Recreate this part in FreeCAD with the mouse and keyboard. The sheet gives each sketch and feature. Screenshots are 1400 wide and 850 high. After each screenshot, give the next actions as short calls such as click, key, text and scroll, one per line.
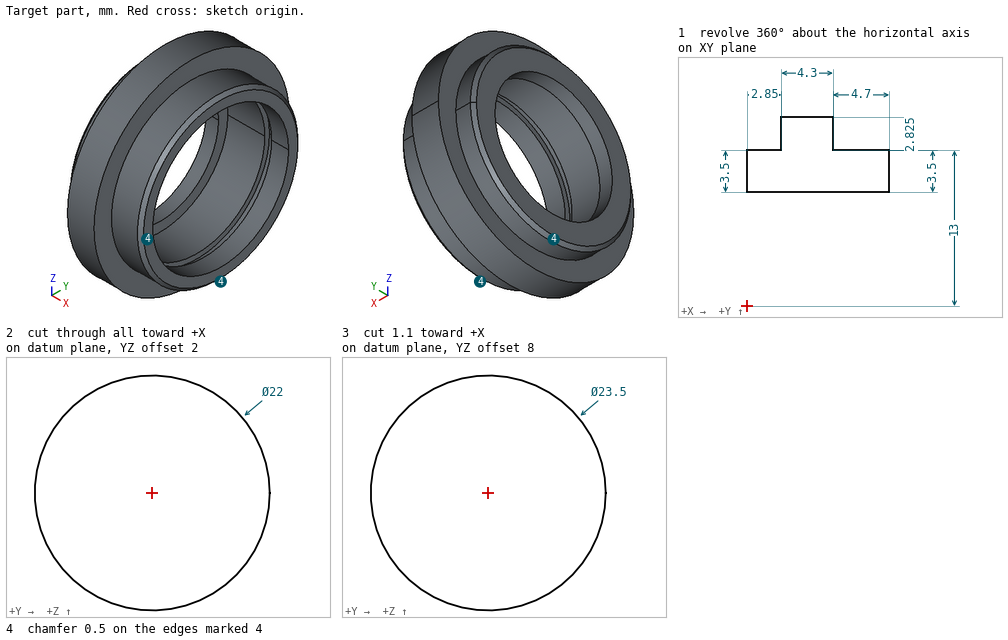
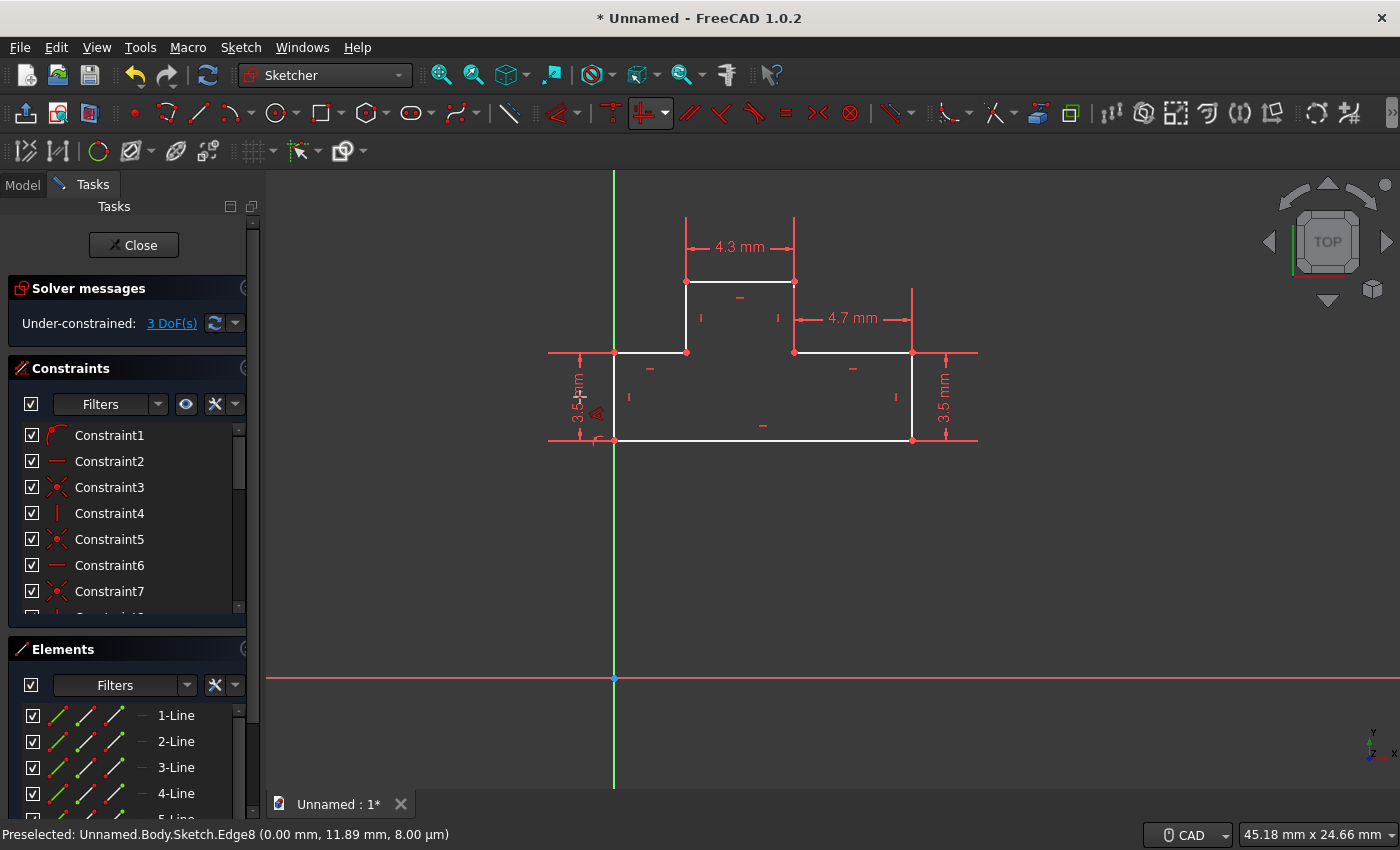
click(912, 353)
click(946, 516)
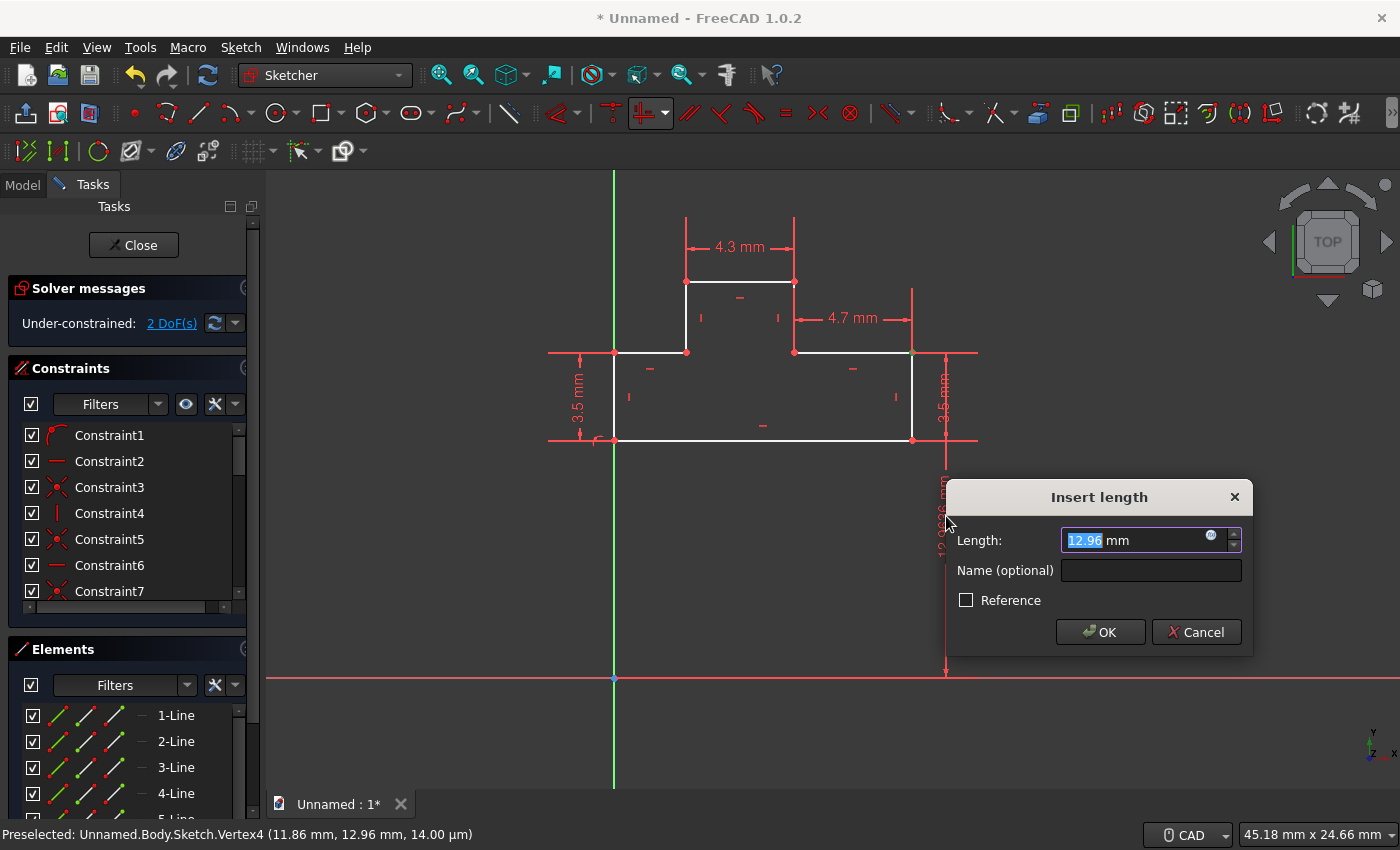
text(13)
key(Return)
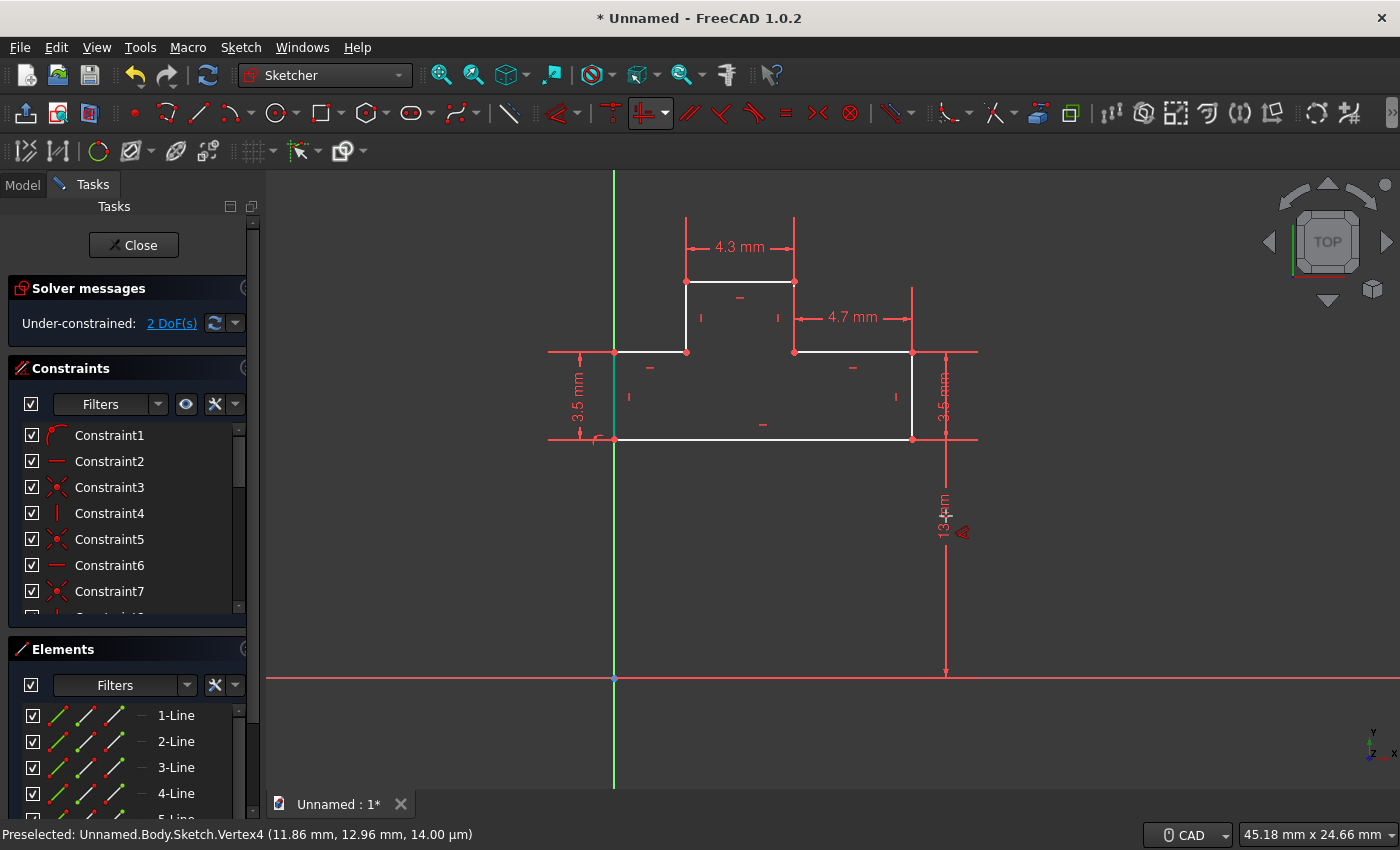
click(665, 352)
click(650, 318)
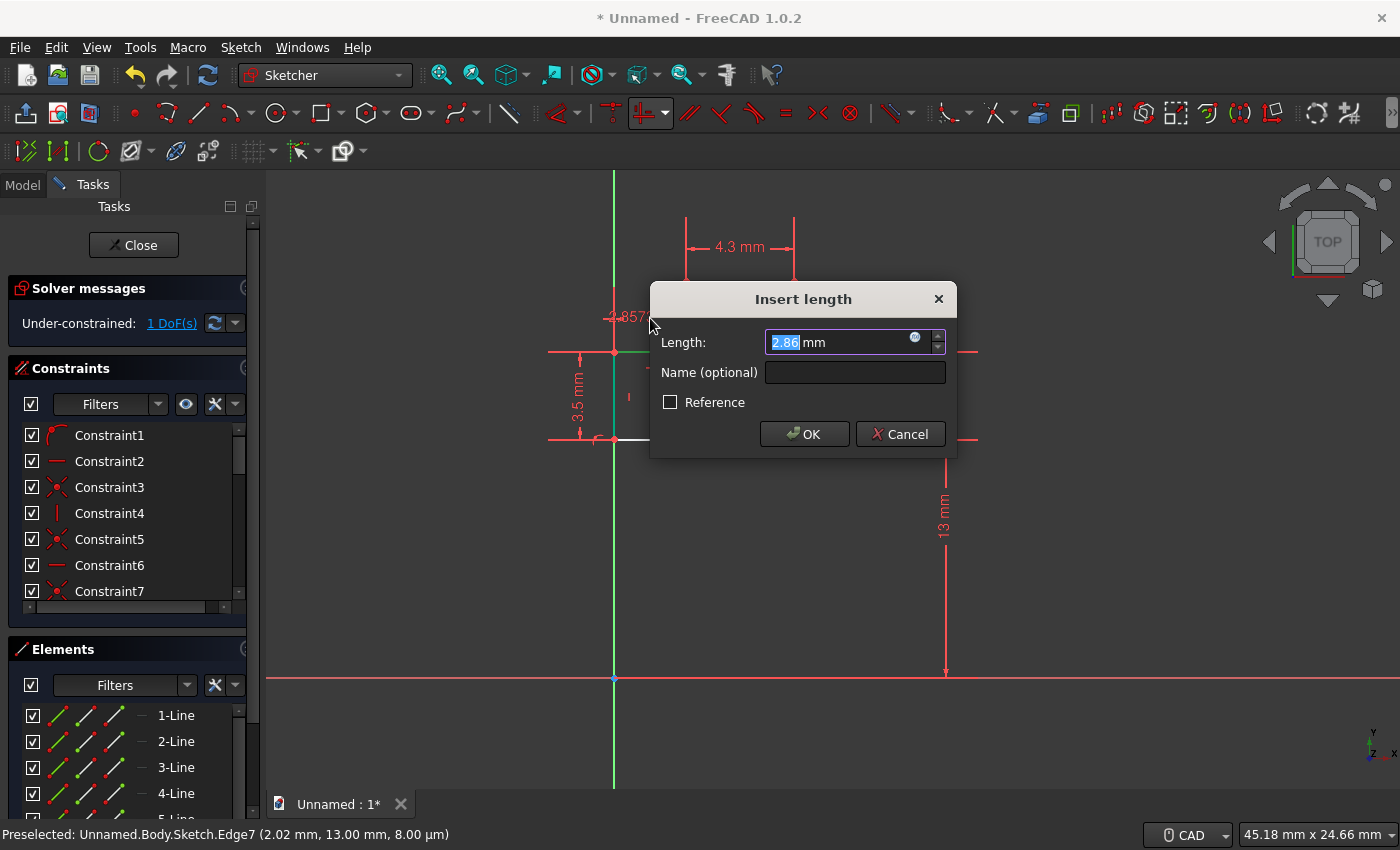
text(2.85)
key(Return)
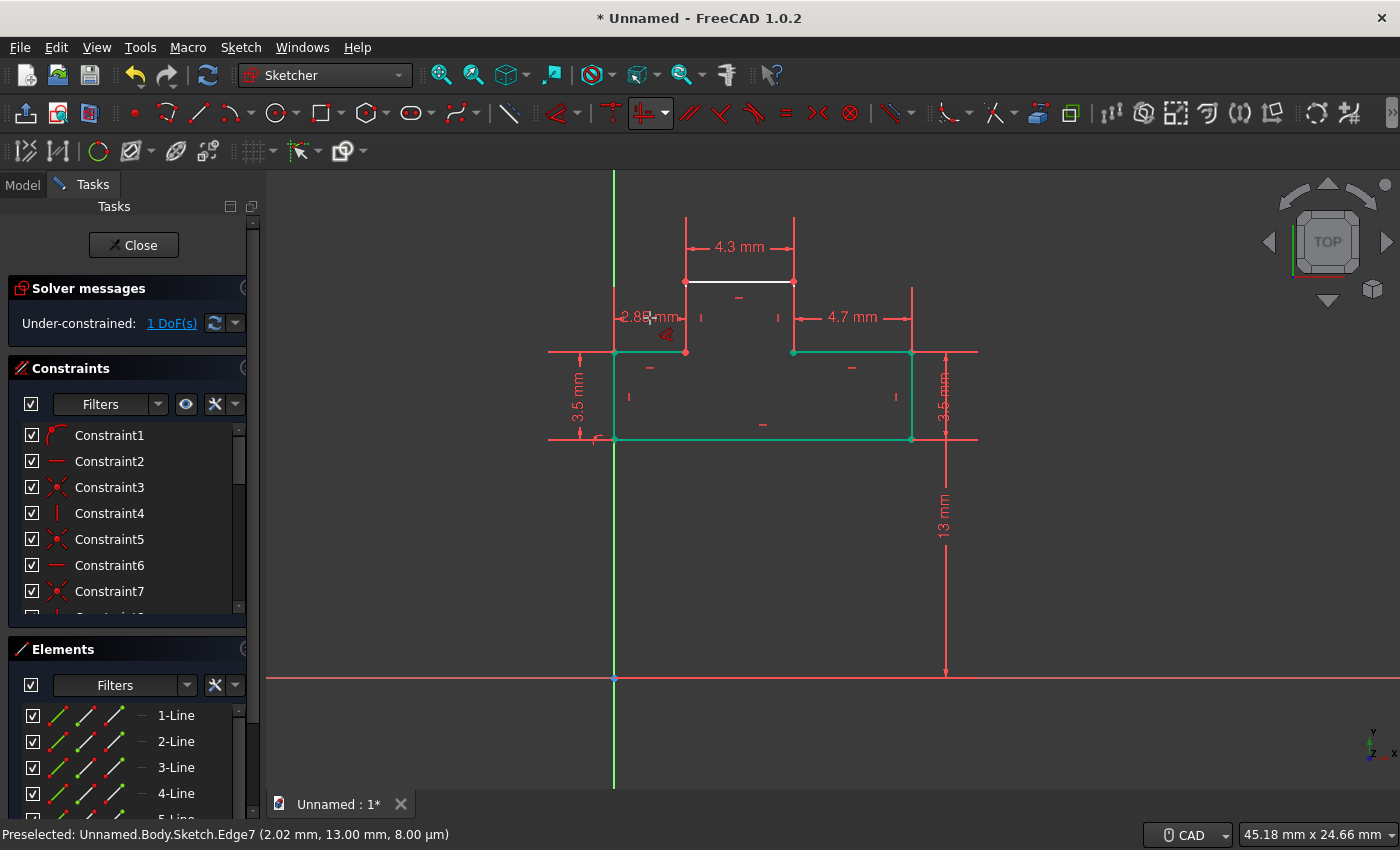
click(794, 331)
click(828, 293)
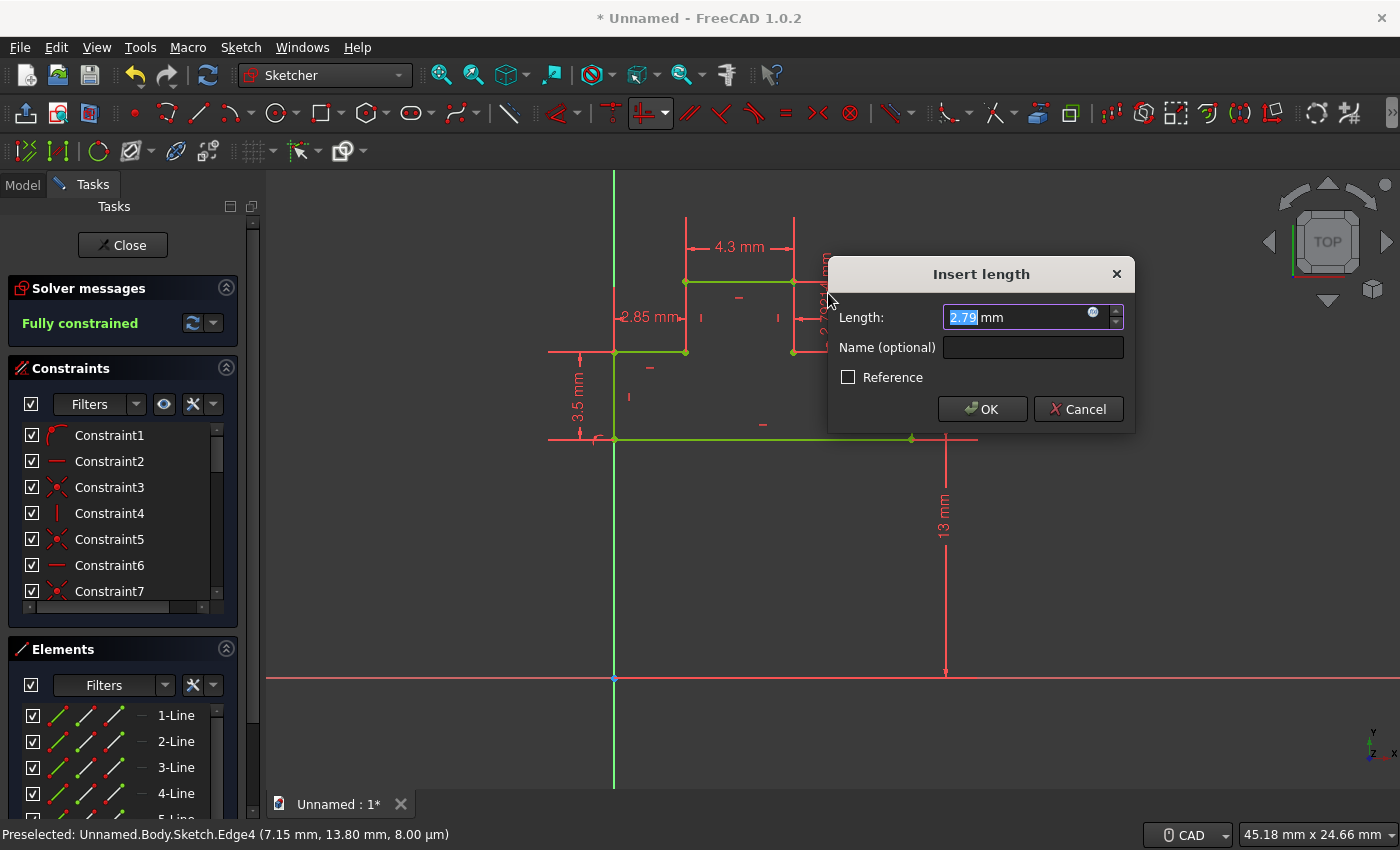
text(2.825)
key(Return)
key(Escape)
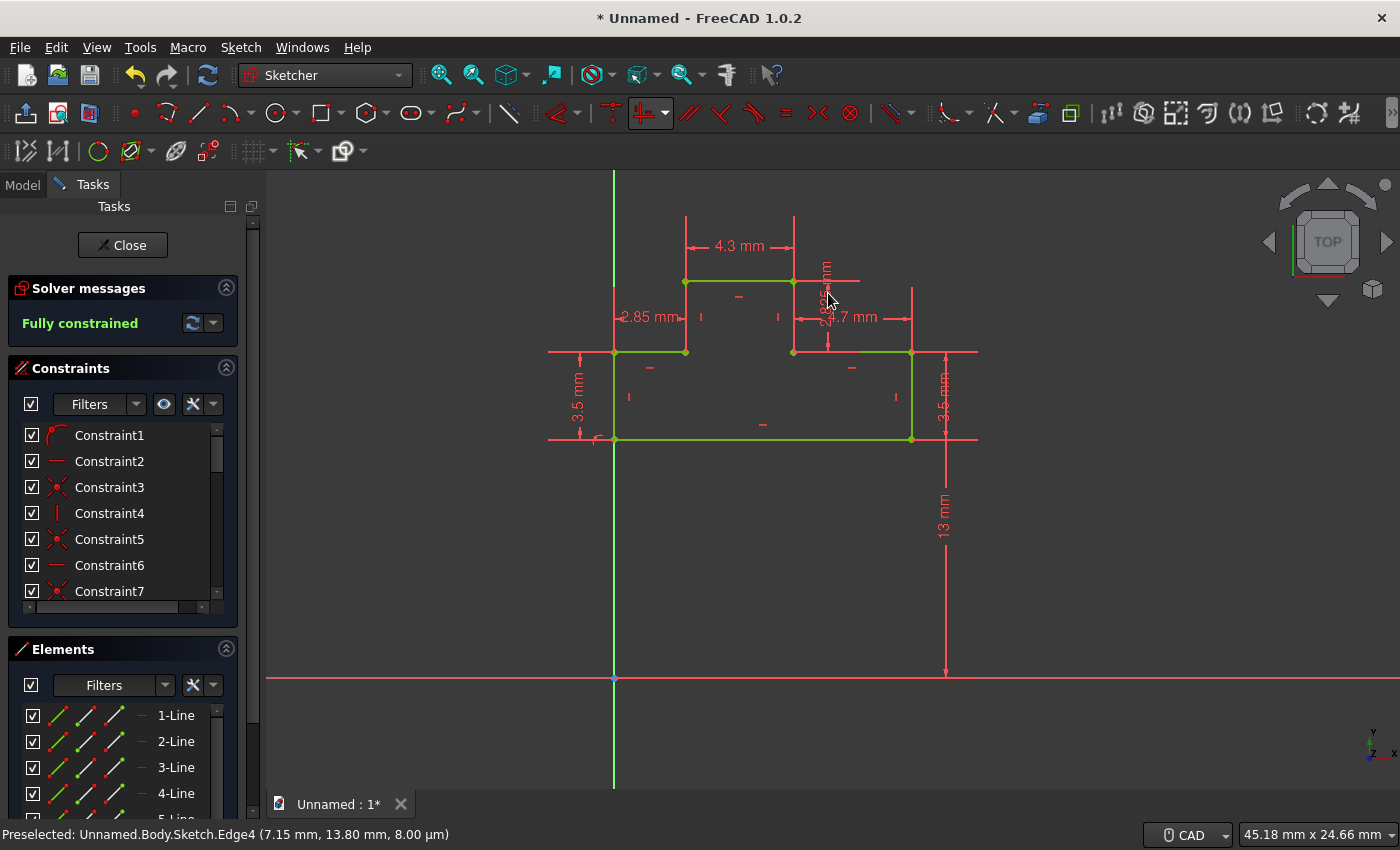
click(123, 245)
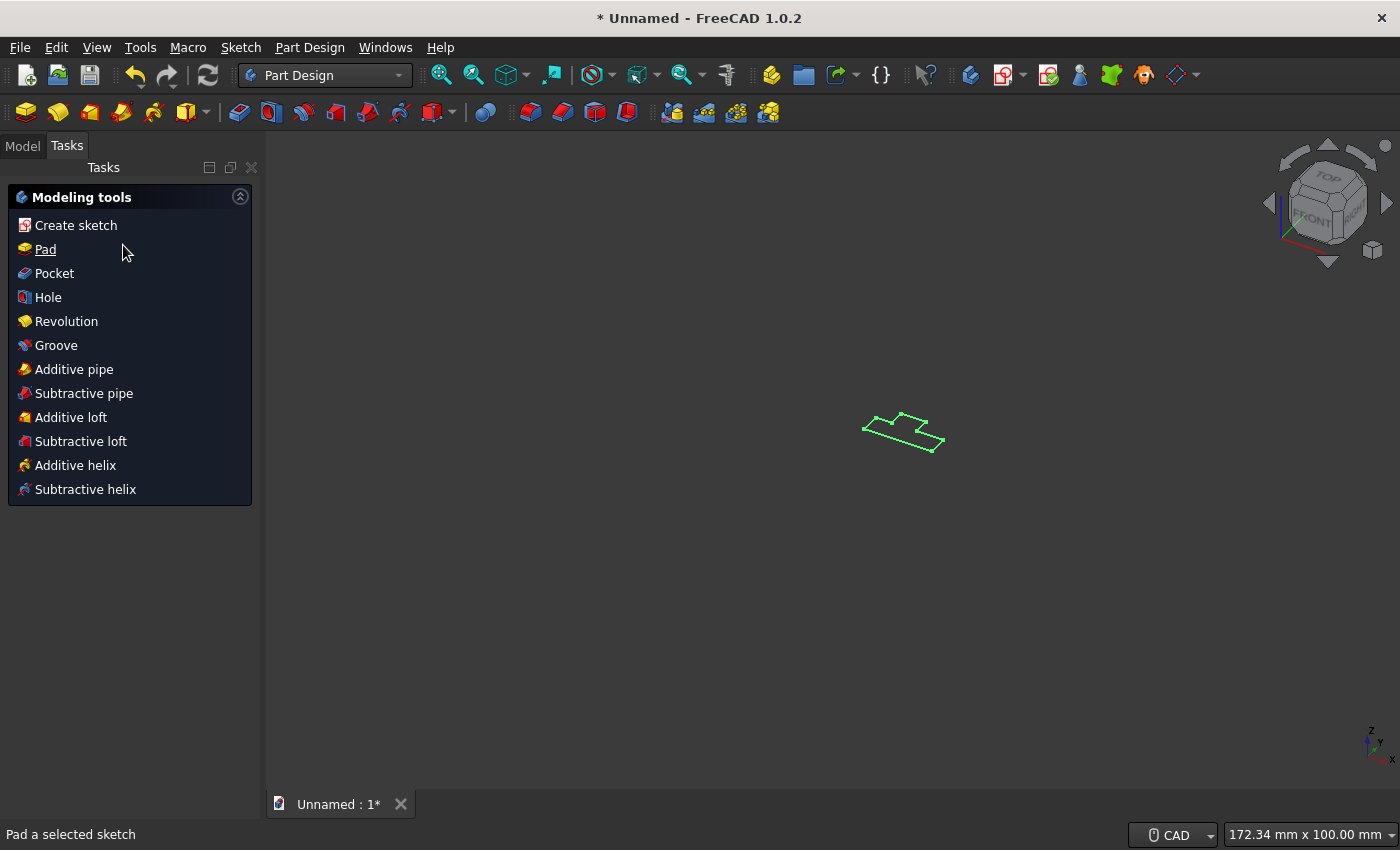
click(58, 112)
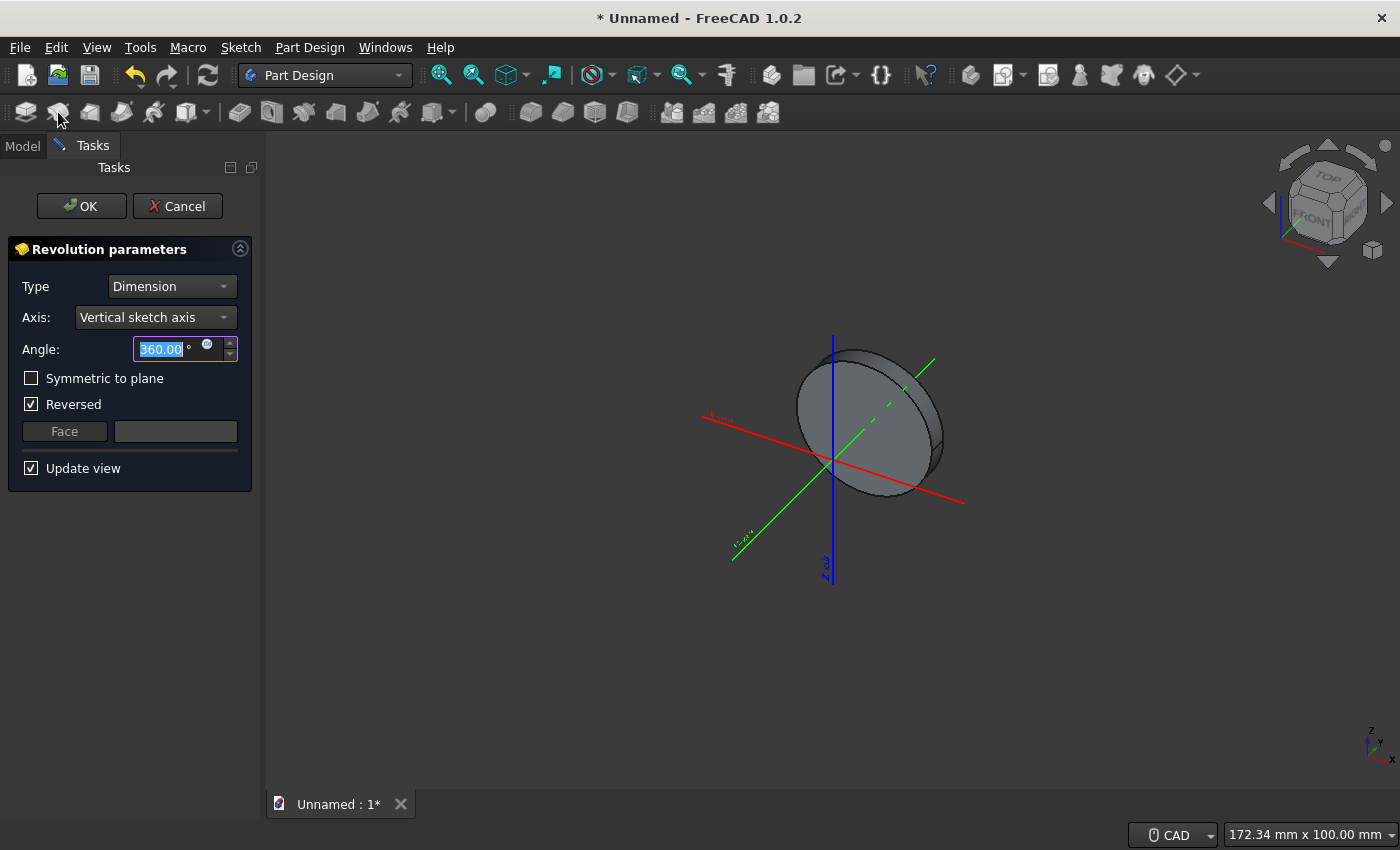
click(156, 318)